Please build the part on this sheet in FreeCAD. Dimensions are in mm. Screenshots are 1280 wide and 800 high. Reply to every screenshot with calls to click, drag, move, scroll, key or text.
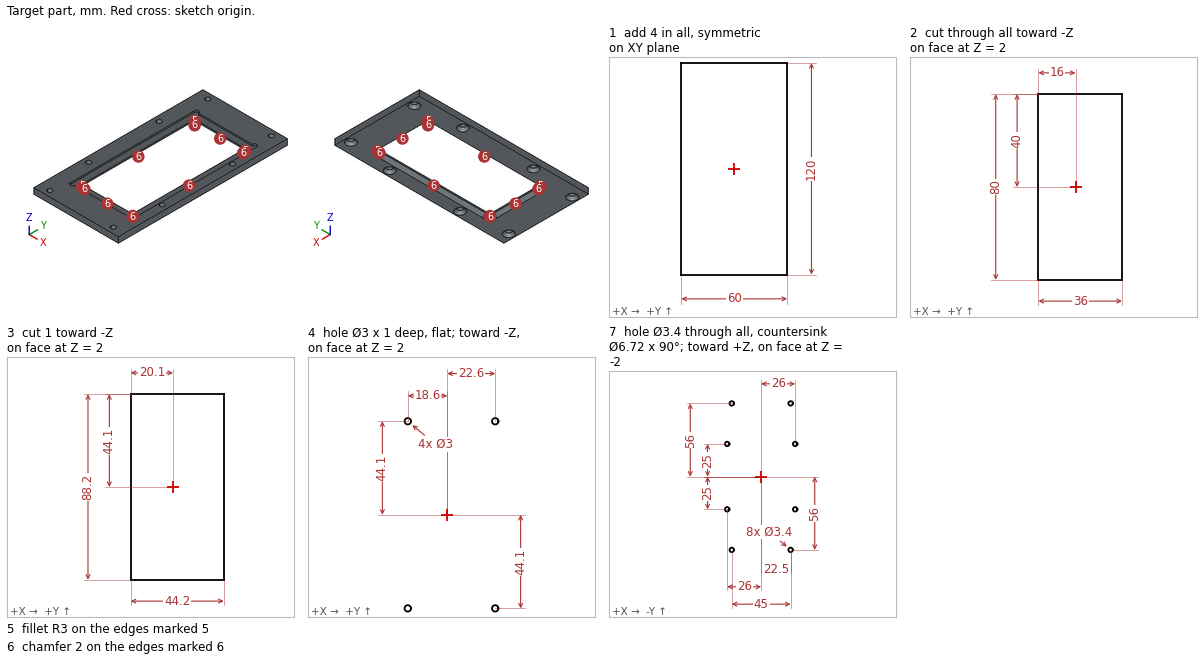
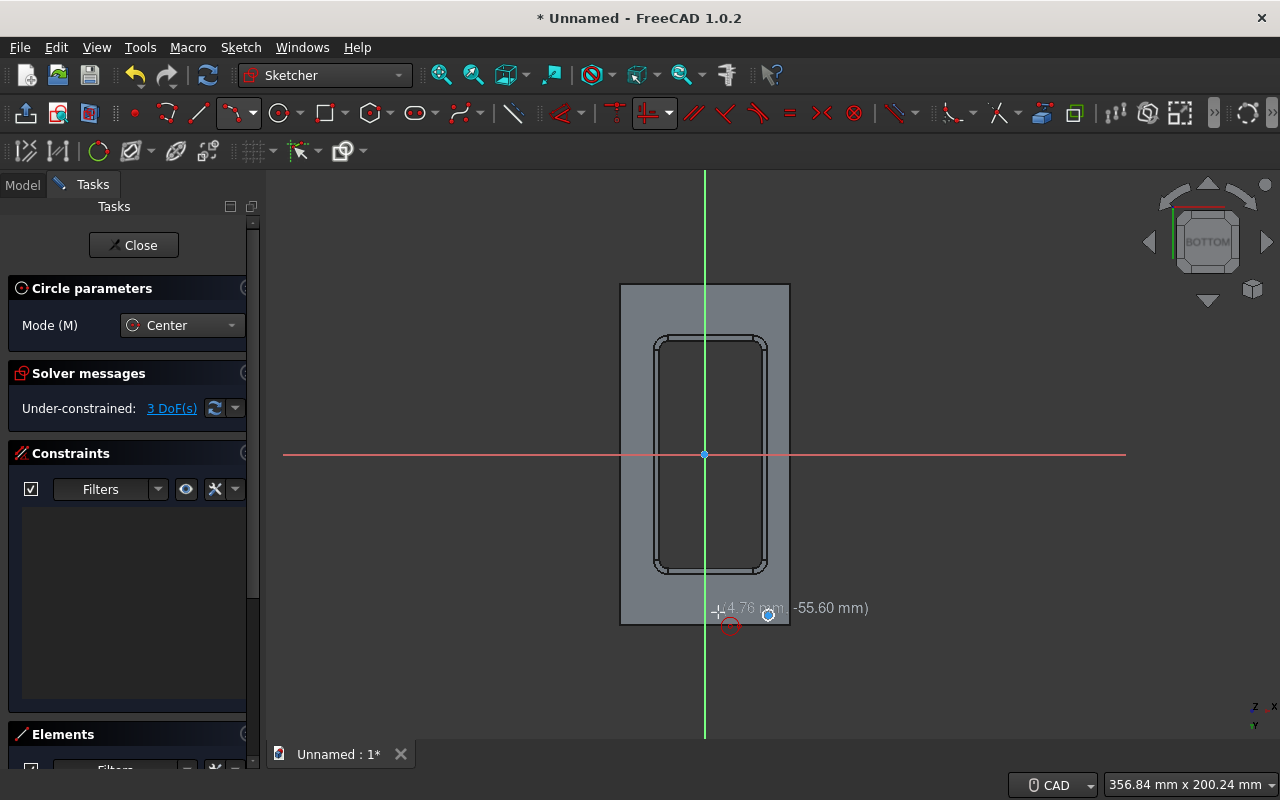
click(641, 614)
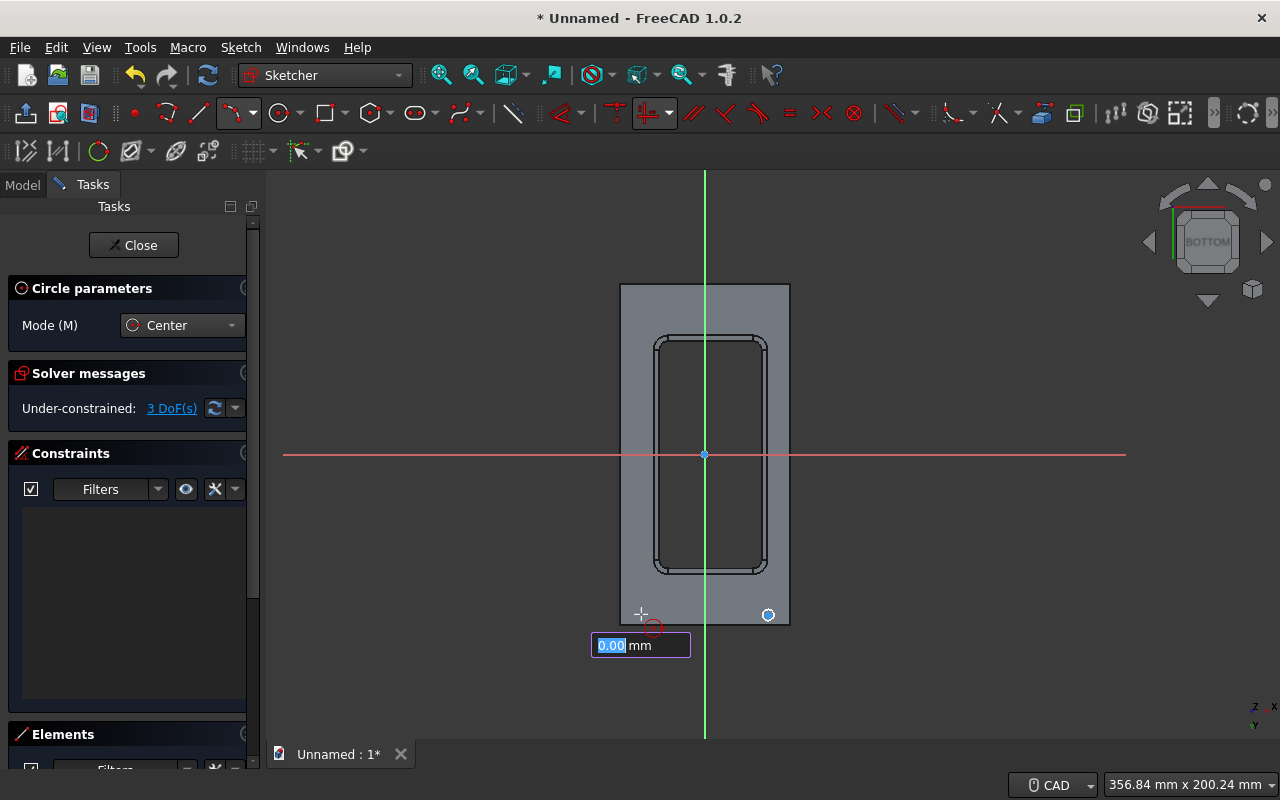
scroll(644, 611, up, 6)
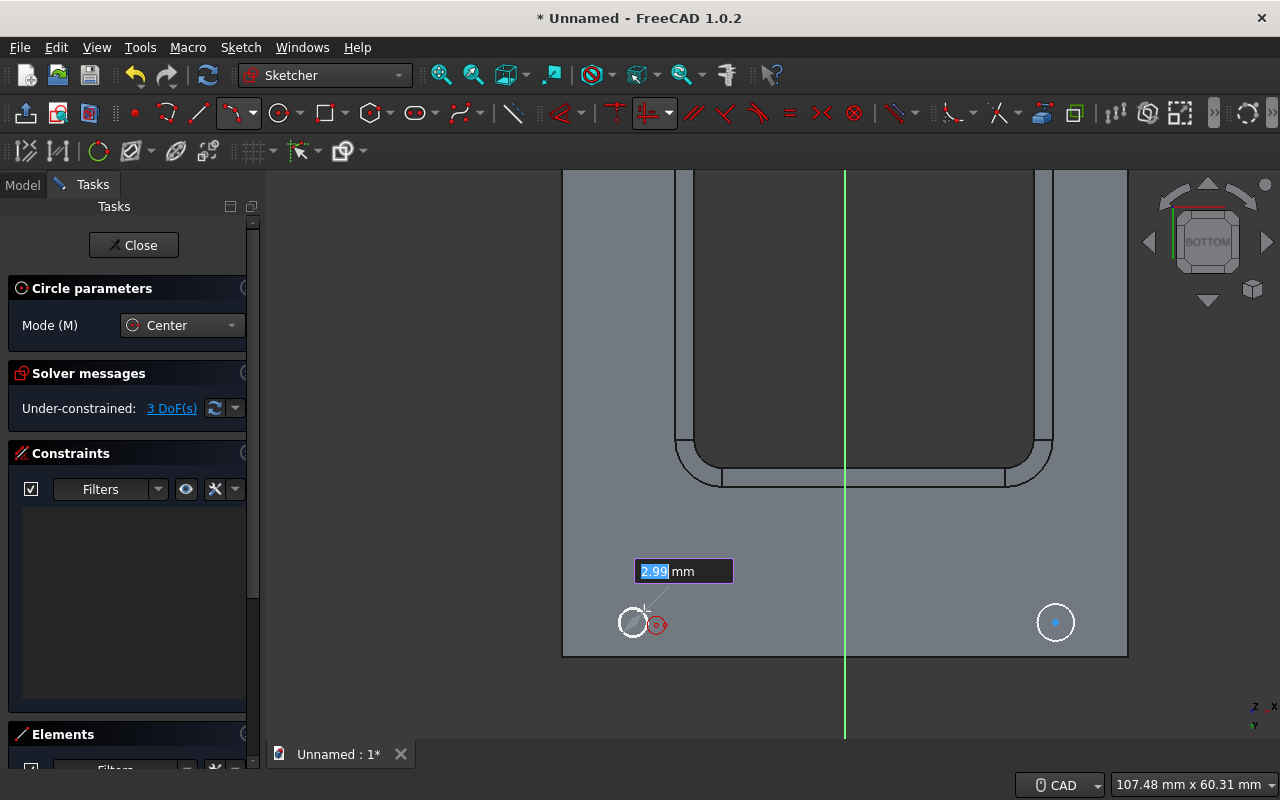
click(644, 608)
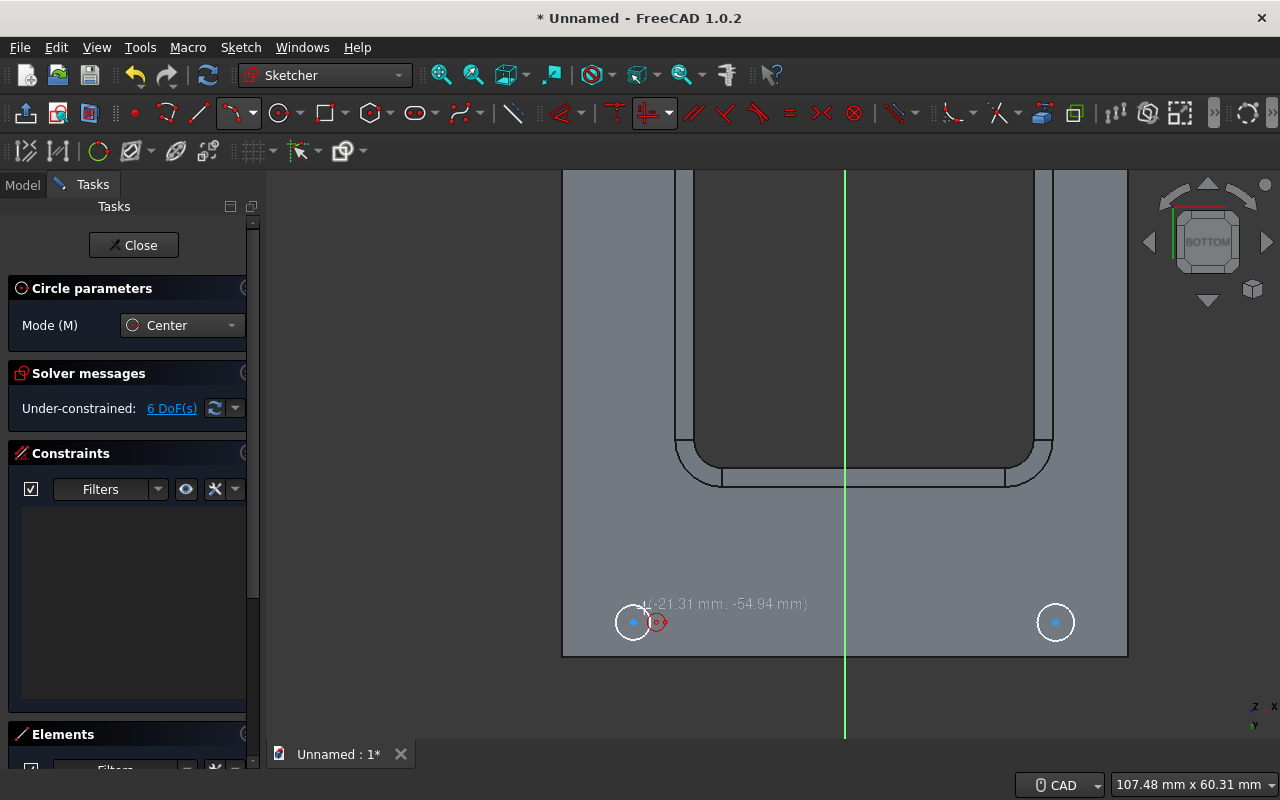
scroll(600, 327, up, 2)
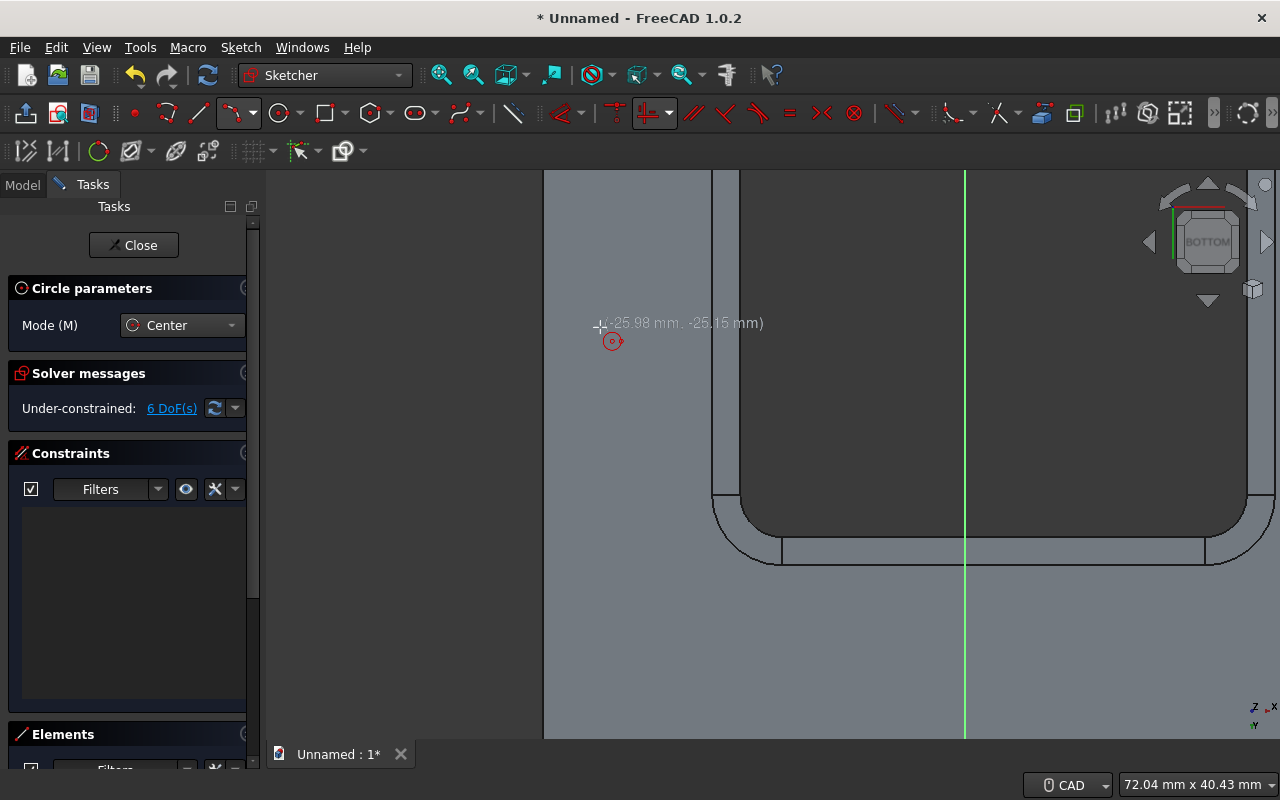
scroll(638, 576, down, 8)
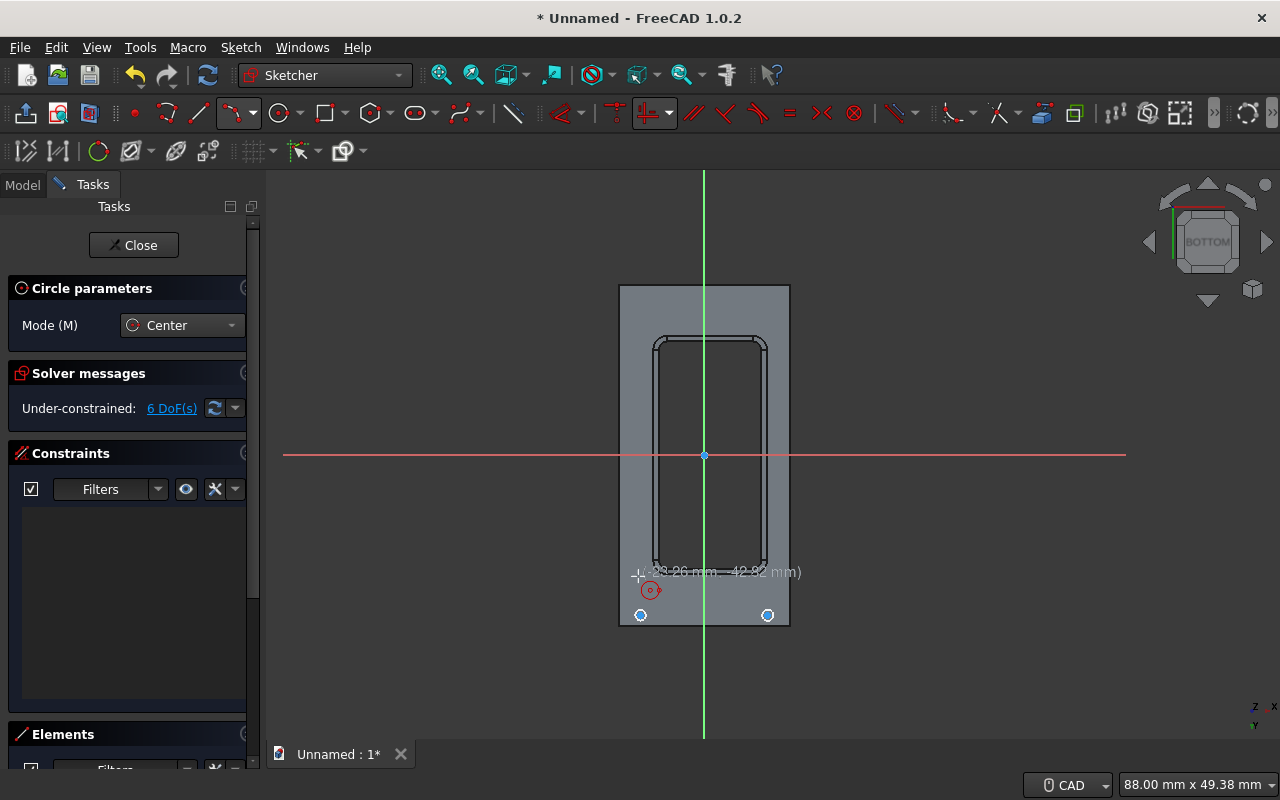
click(631, 526)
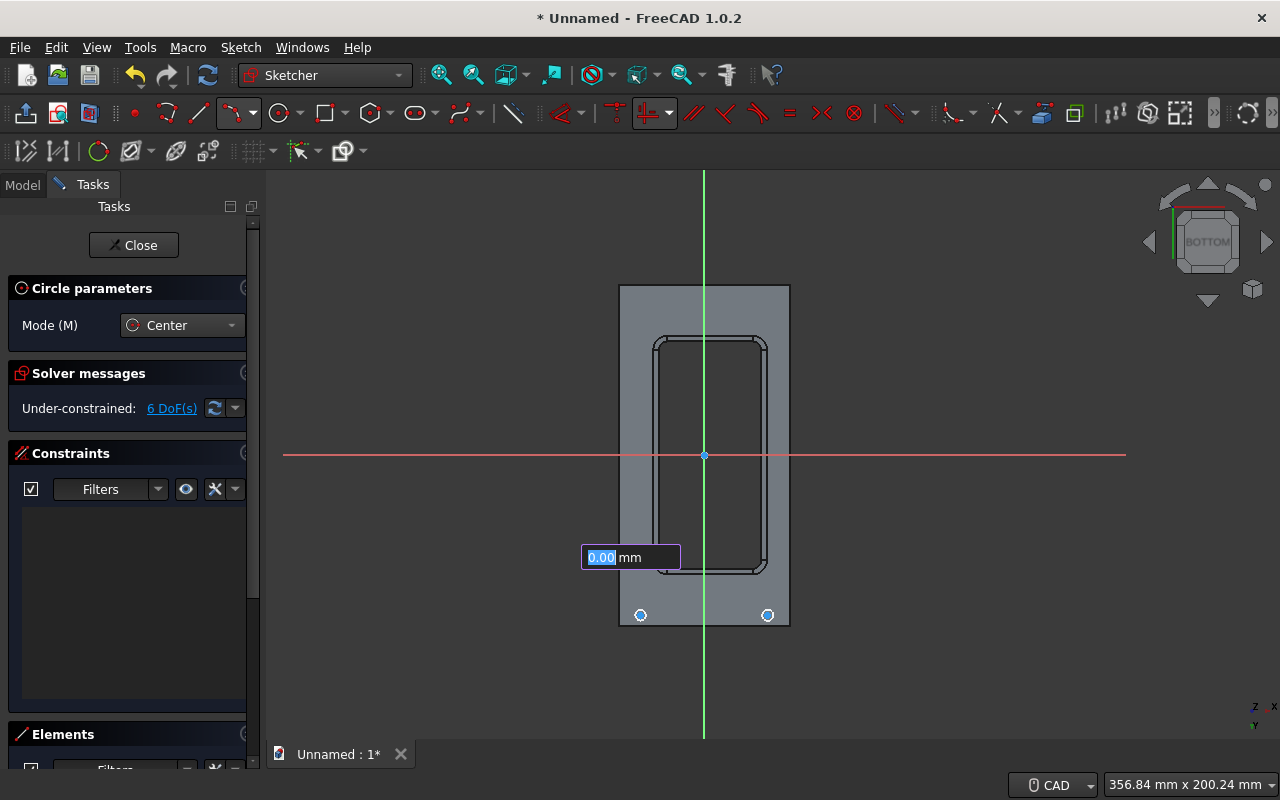
scroll(634, 523, up, 6)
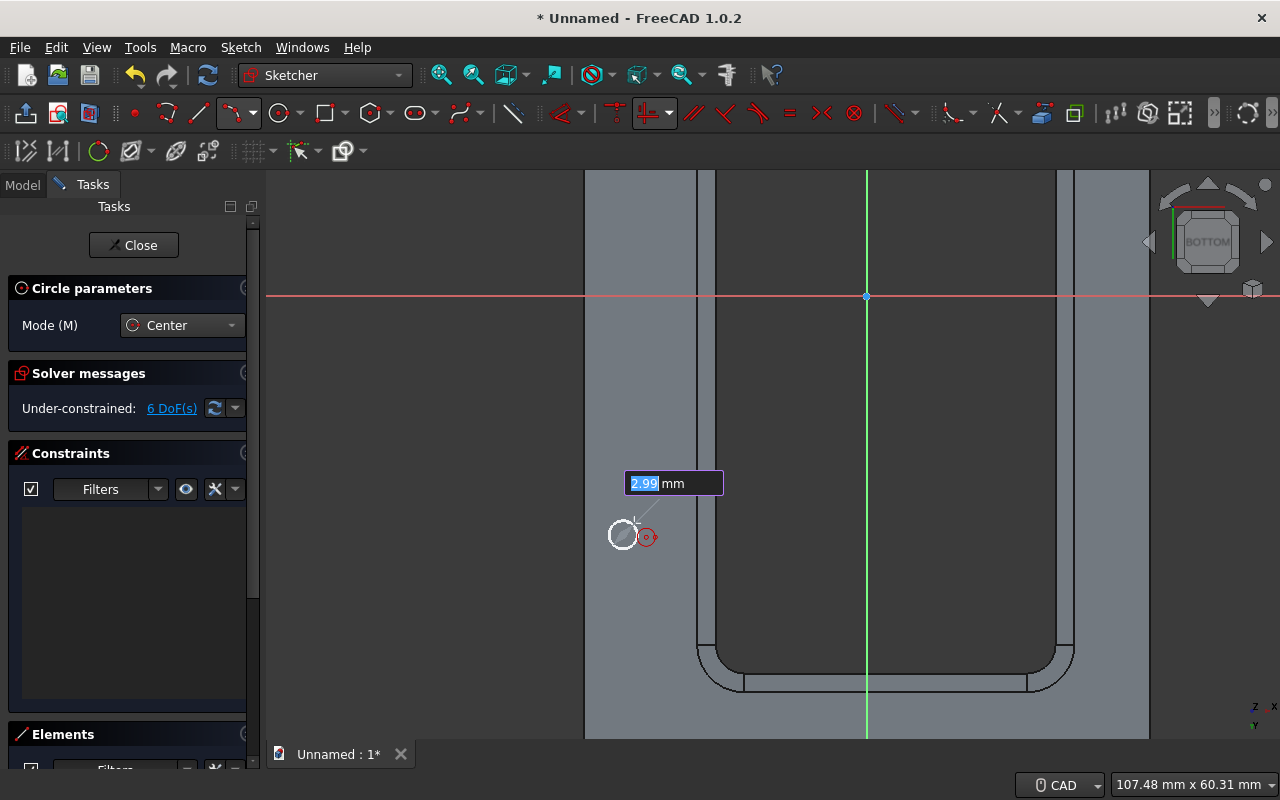
click(633, 521)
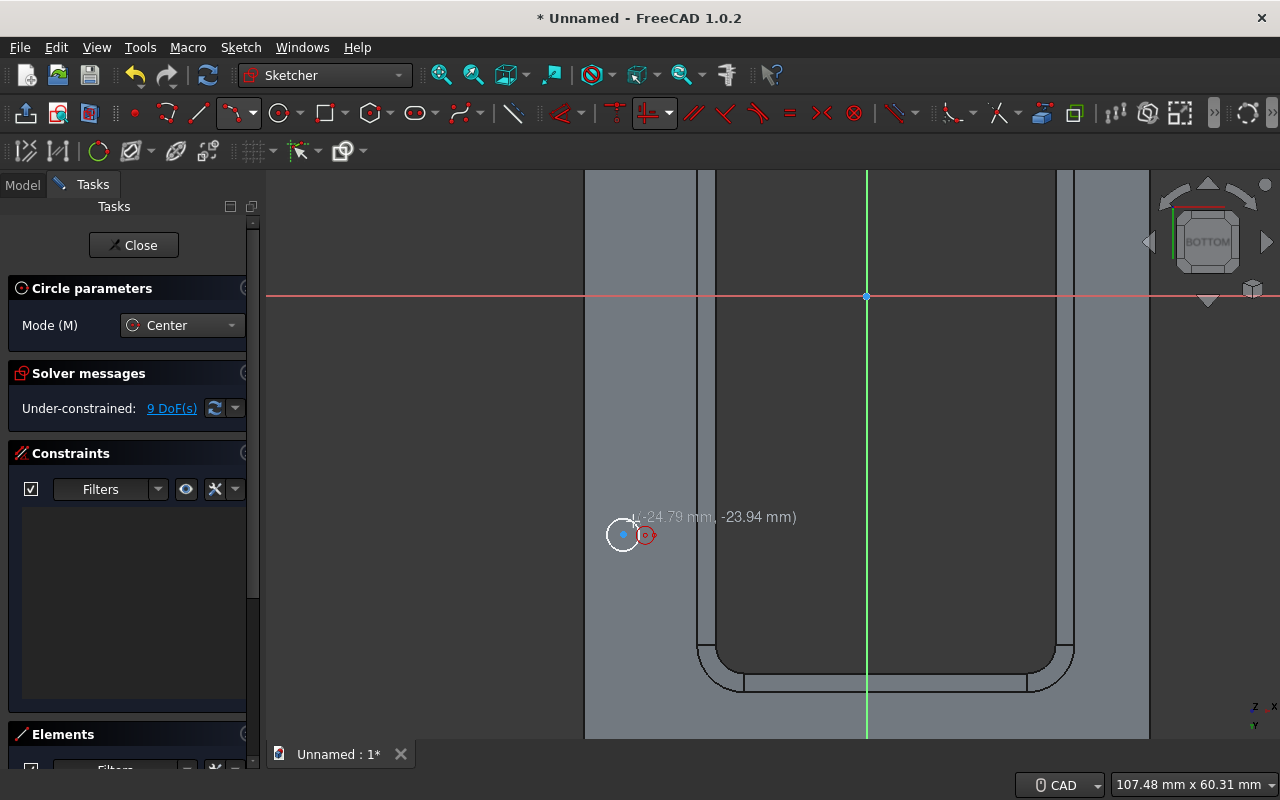
scroll(635, 523, down, 6)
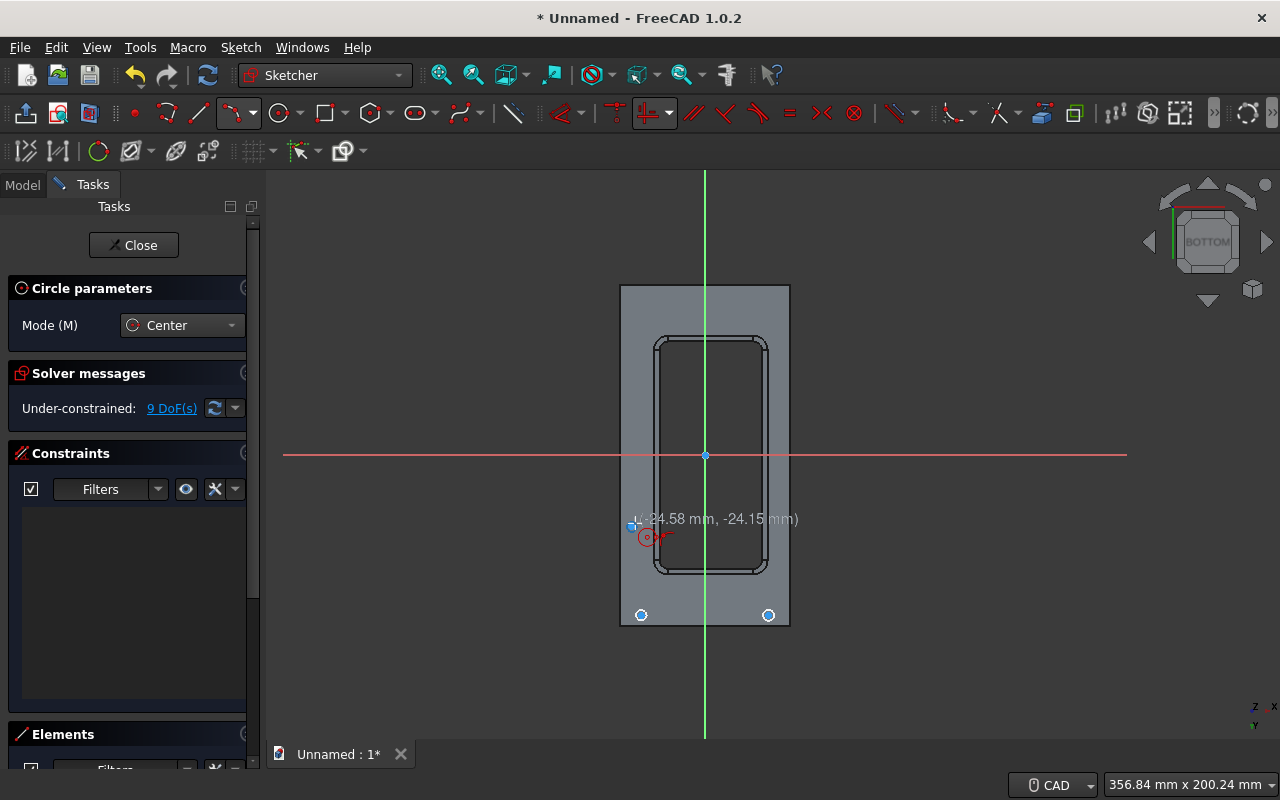
scroll(631, 384, up, 8)